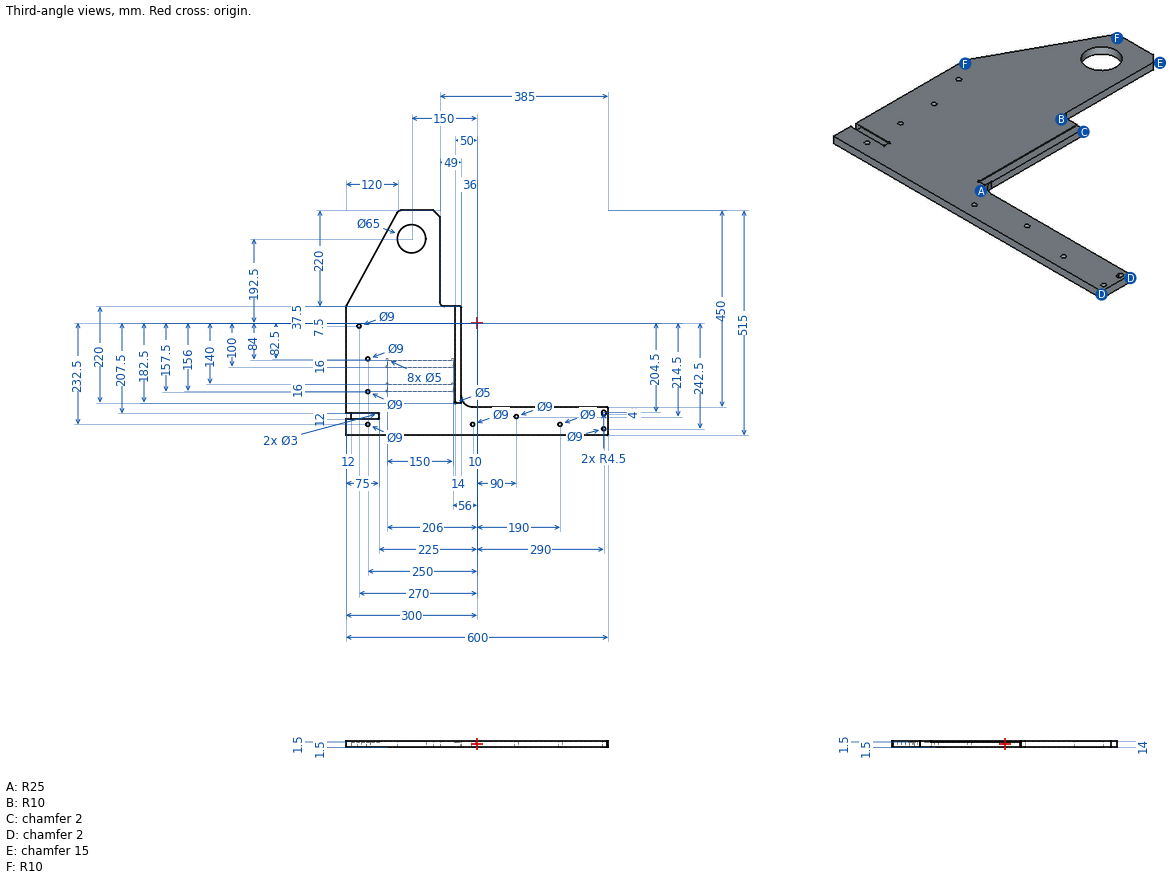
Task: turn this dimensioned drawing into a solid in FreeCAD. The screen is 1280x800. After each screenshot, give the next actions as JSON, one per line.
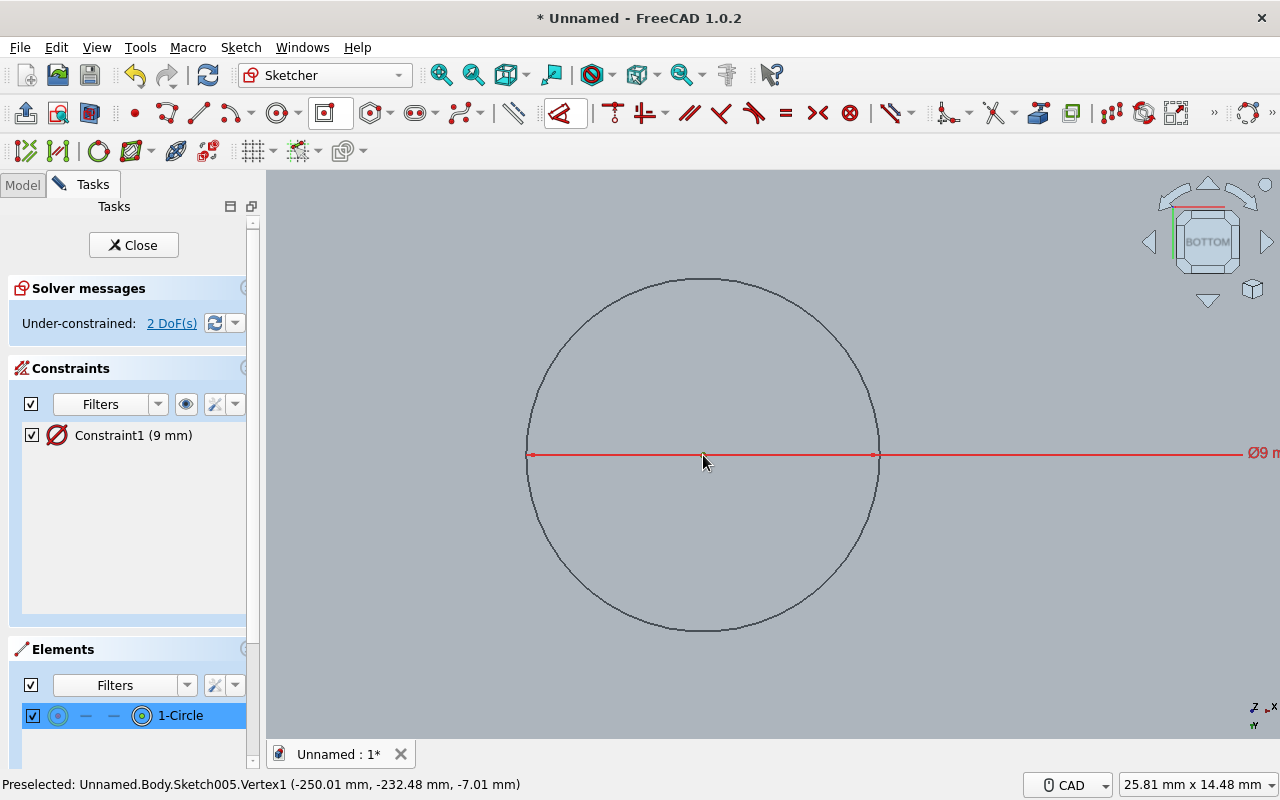
{"action": "left_click", "coordinate": [582, 114]}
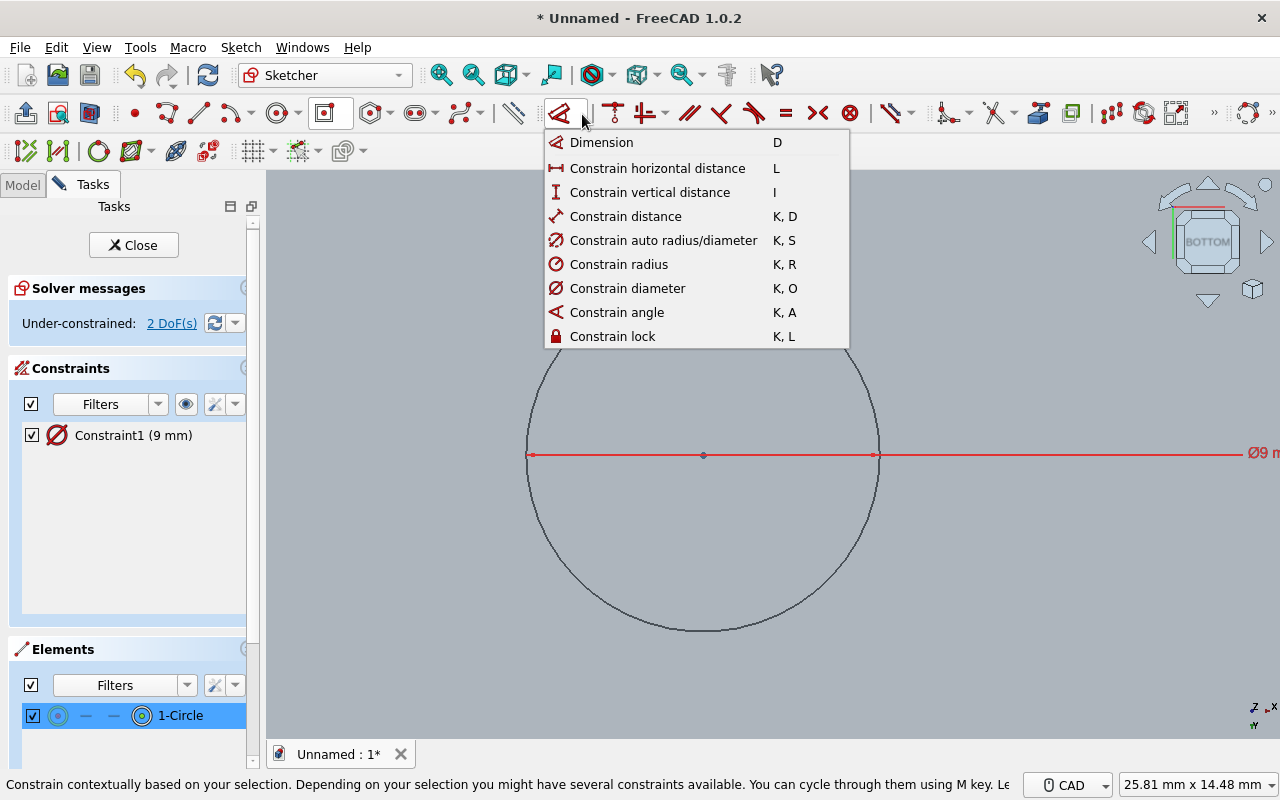
{"action": "left_click", "coordinate": [697, 168]}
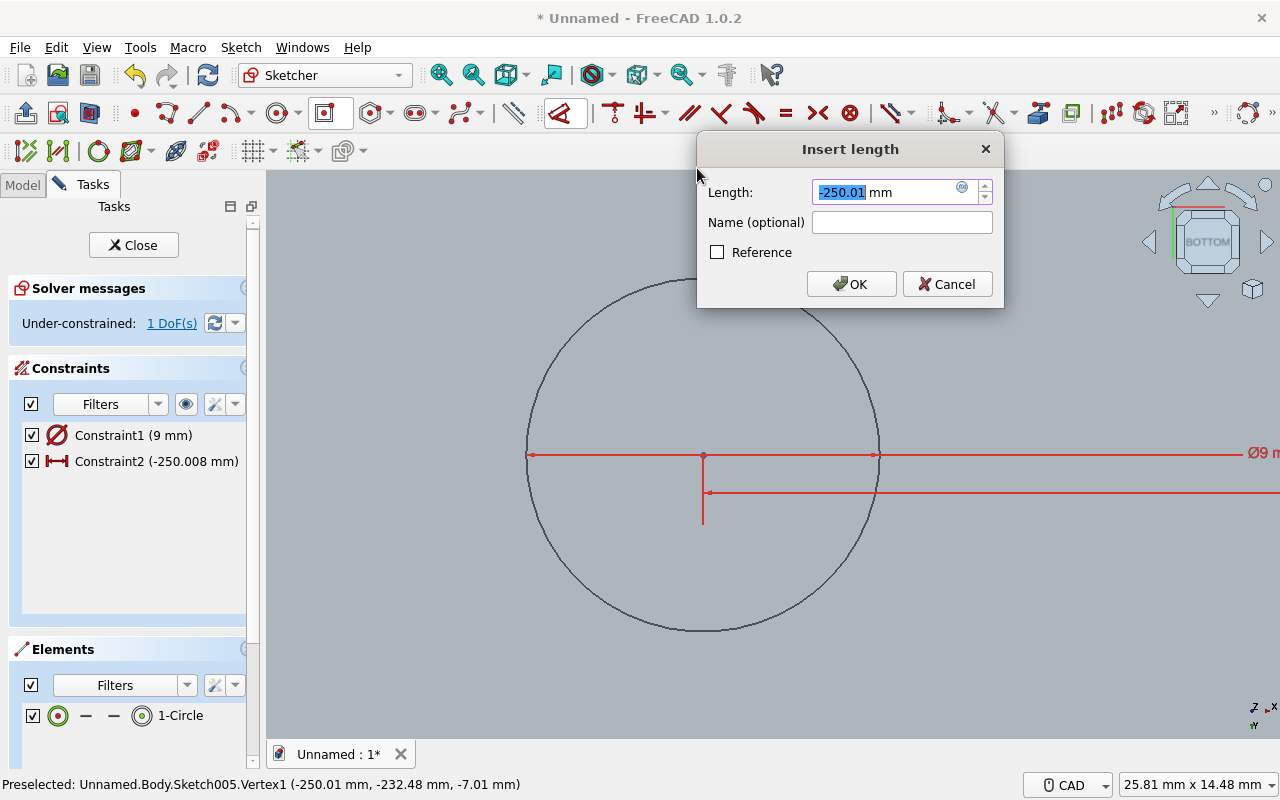
{"action": "type", "text": "-250"}
{"action": "key", "text": "Return"}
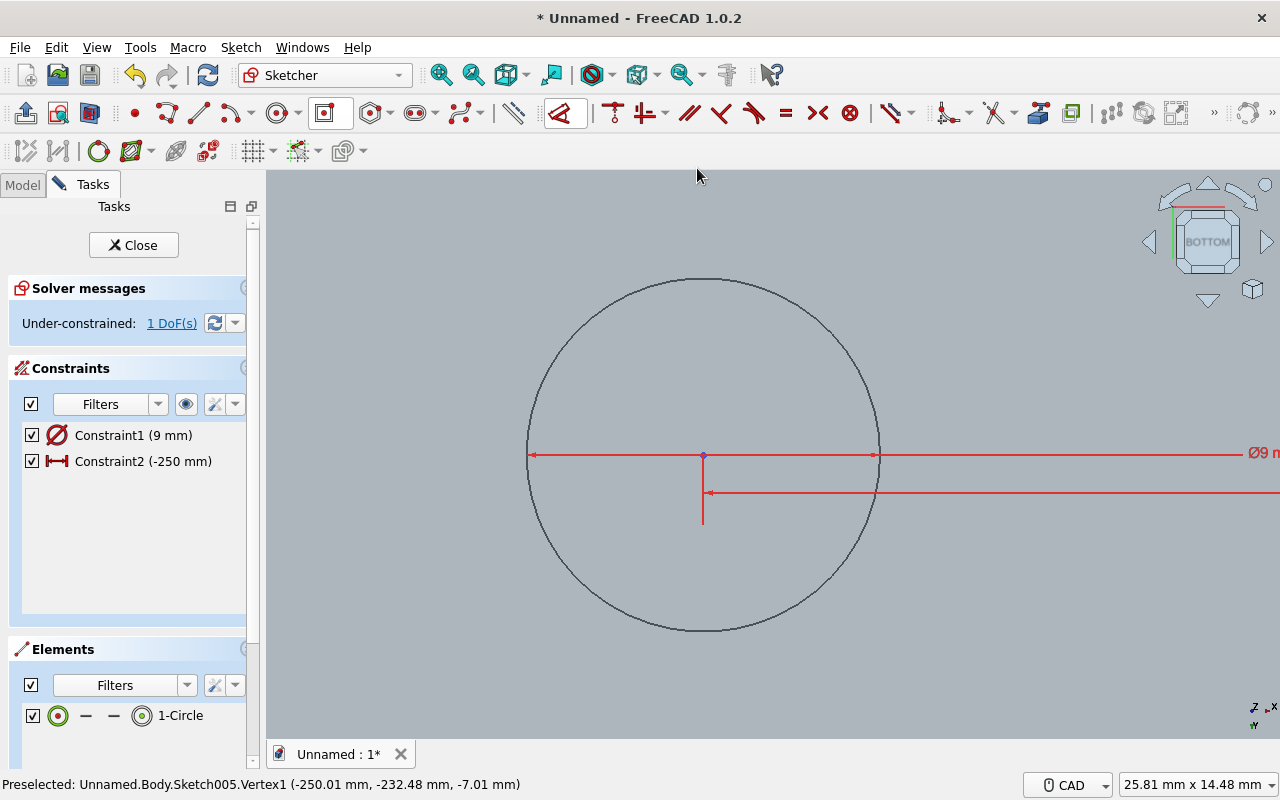
{"action": "left_click", "coordinate": [703, 455]}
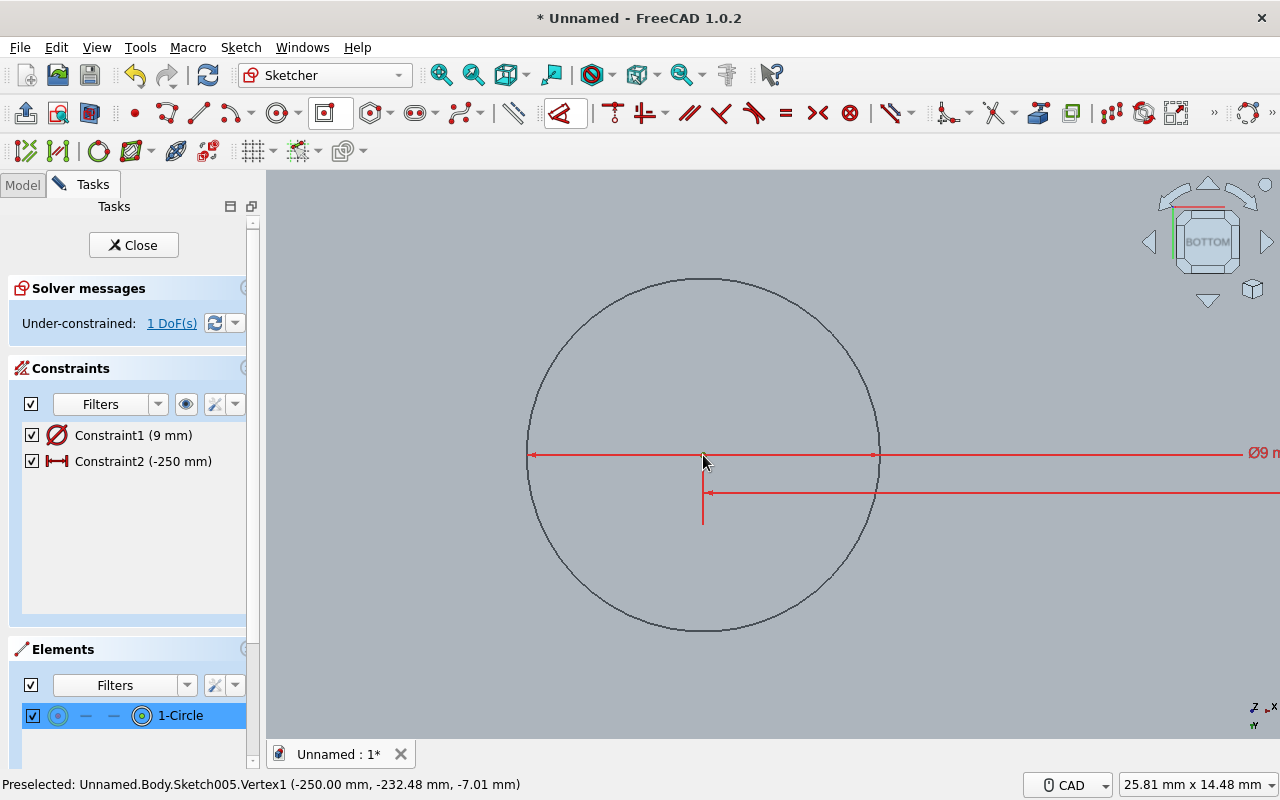
{"action": "key", "text": "i"}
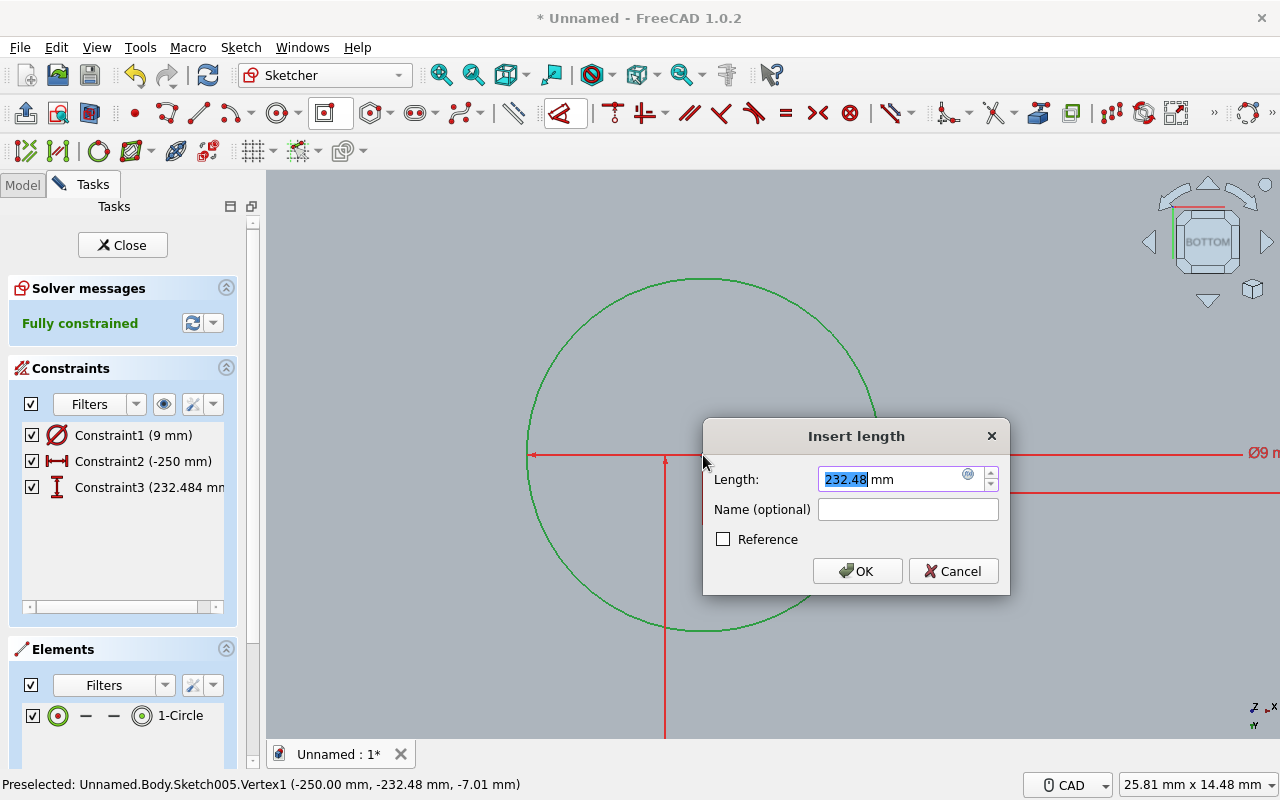
{"action": "type", "text": "232.5"}
{"action": "key", "text": "Return"}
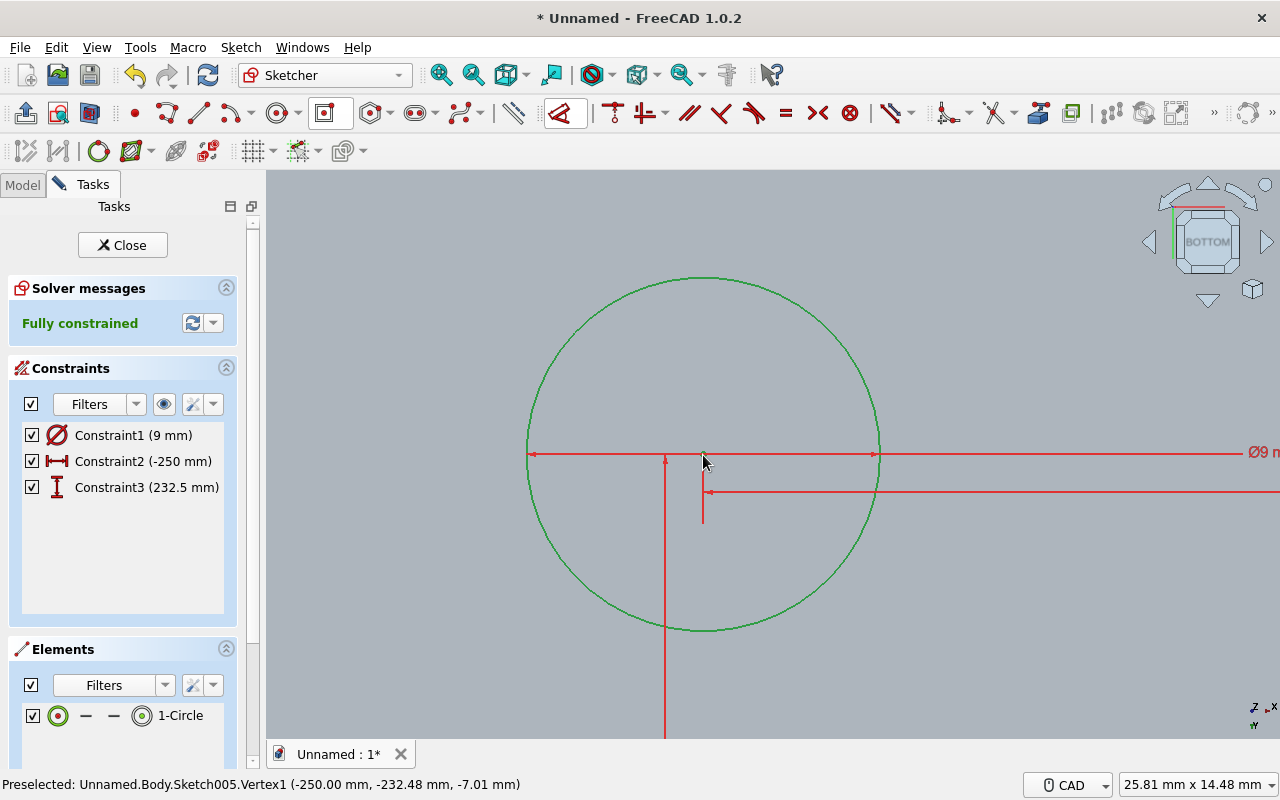
{"action": "left_click", "coordinate": [123, 245]}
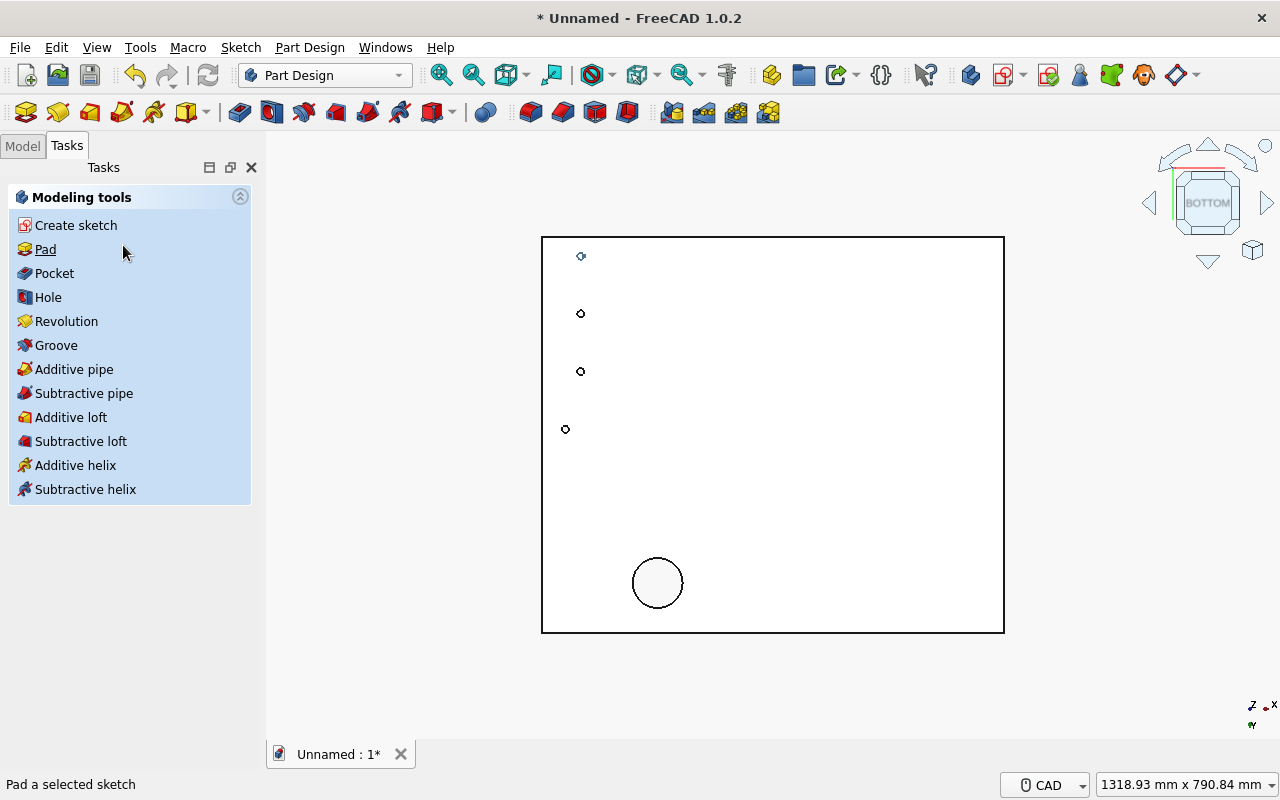
{"action": "left_click", "coordinate": [240, 112]}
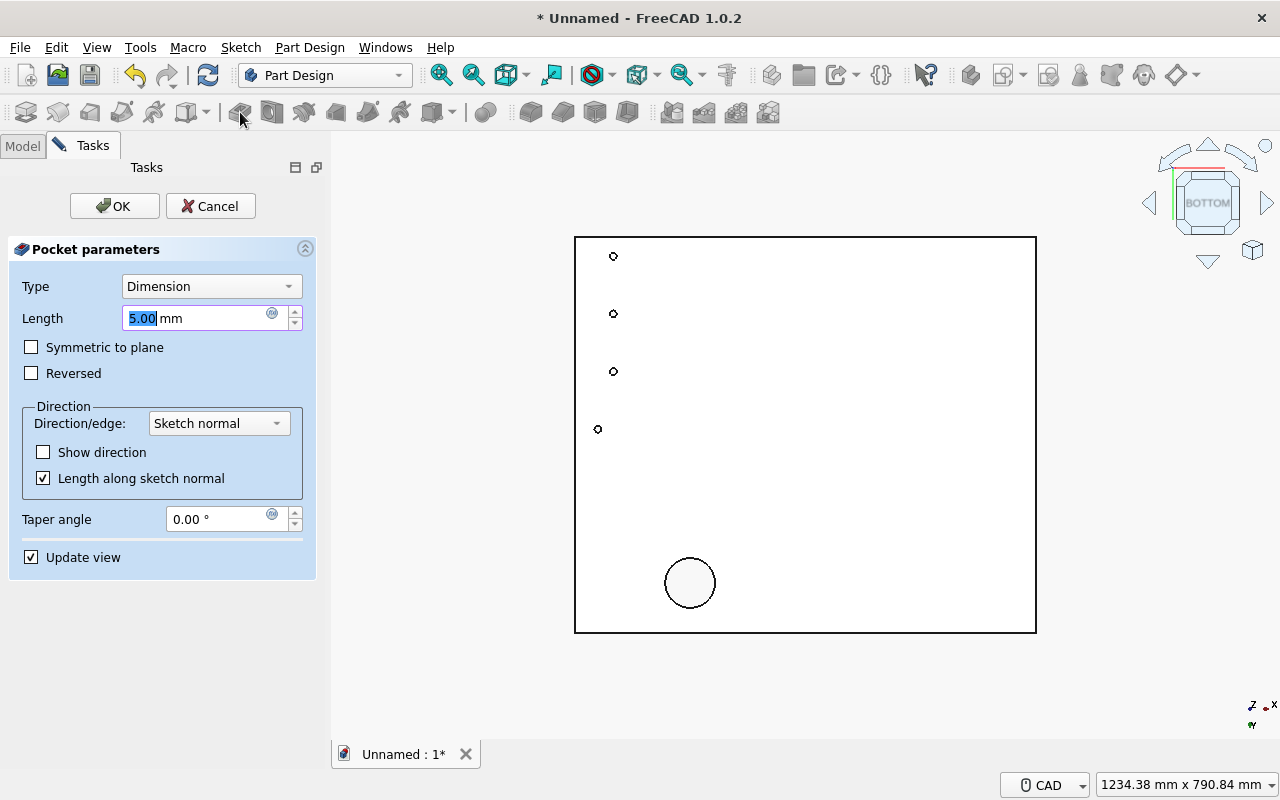
{"action": "left_click", "coordinate": [212, 286]}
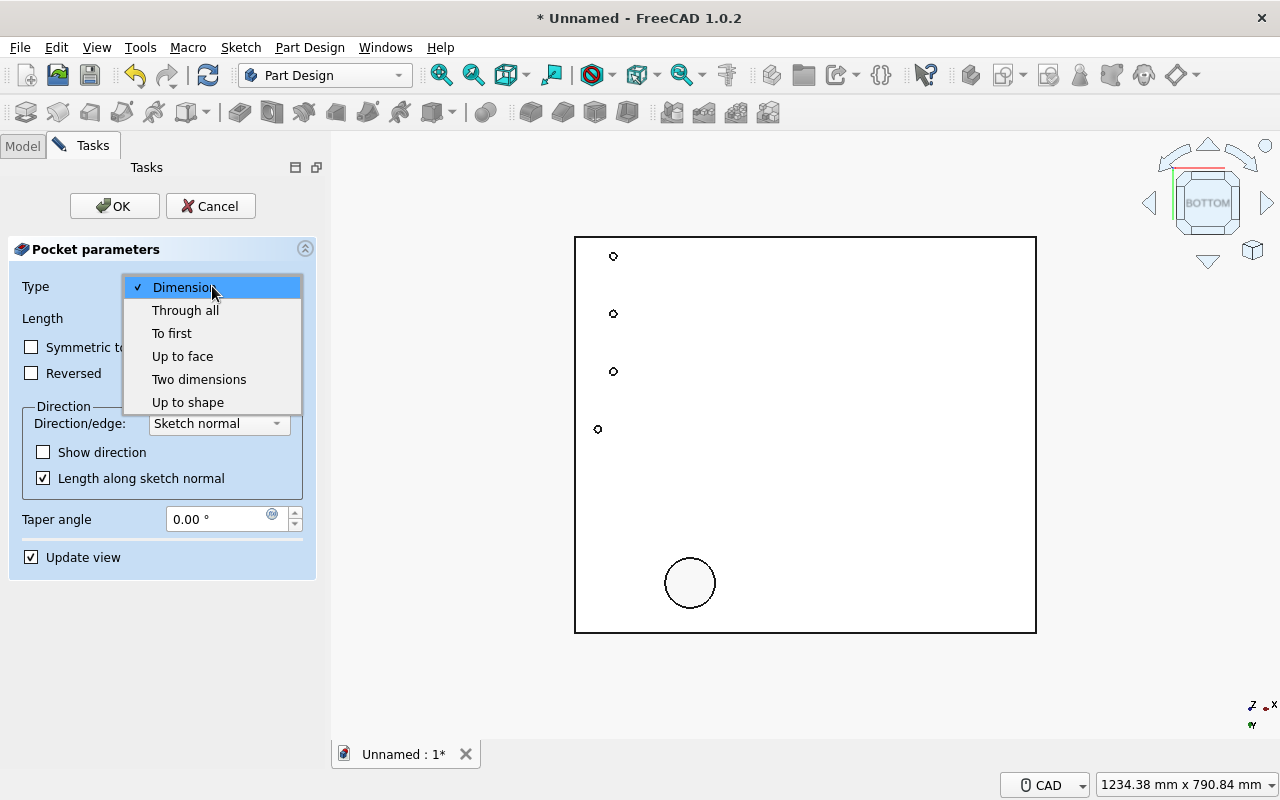
{"action": "left_click", "coordinate": [212, 334]}